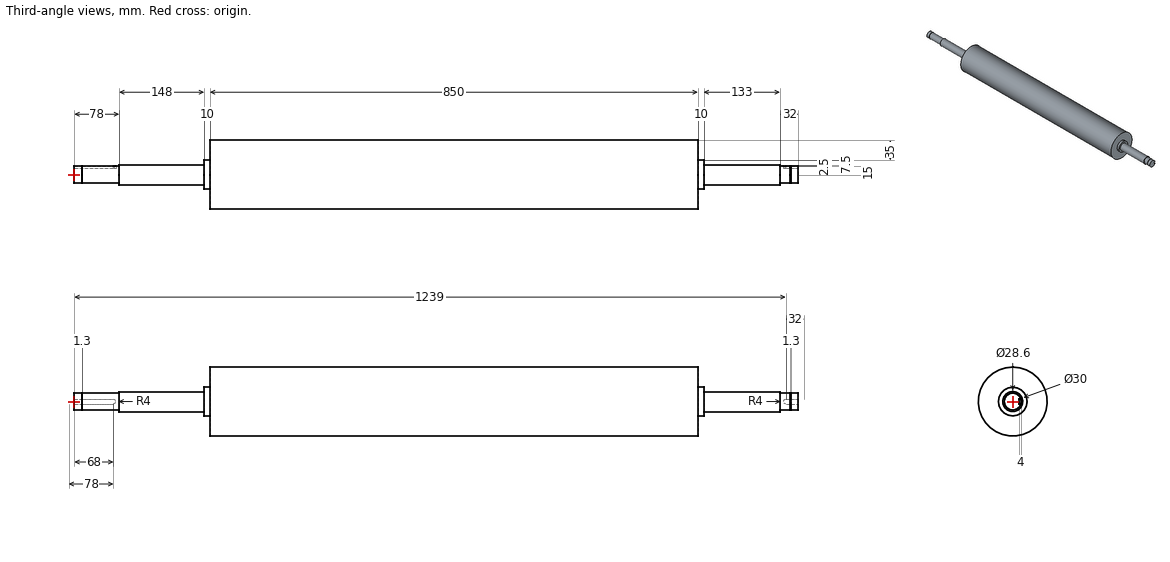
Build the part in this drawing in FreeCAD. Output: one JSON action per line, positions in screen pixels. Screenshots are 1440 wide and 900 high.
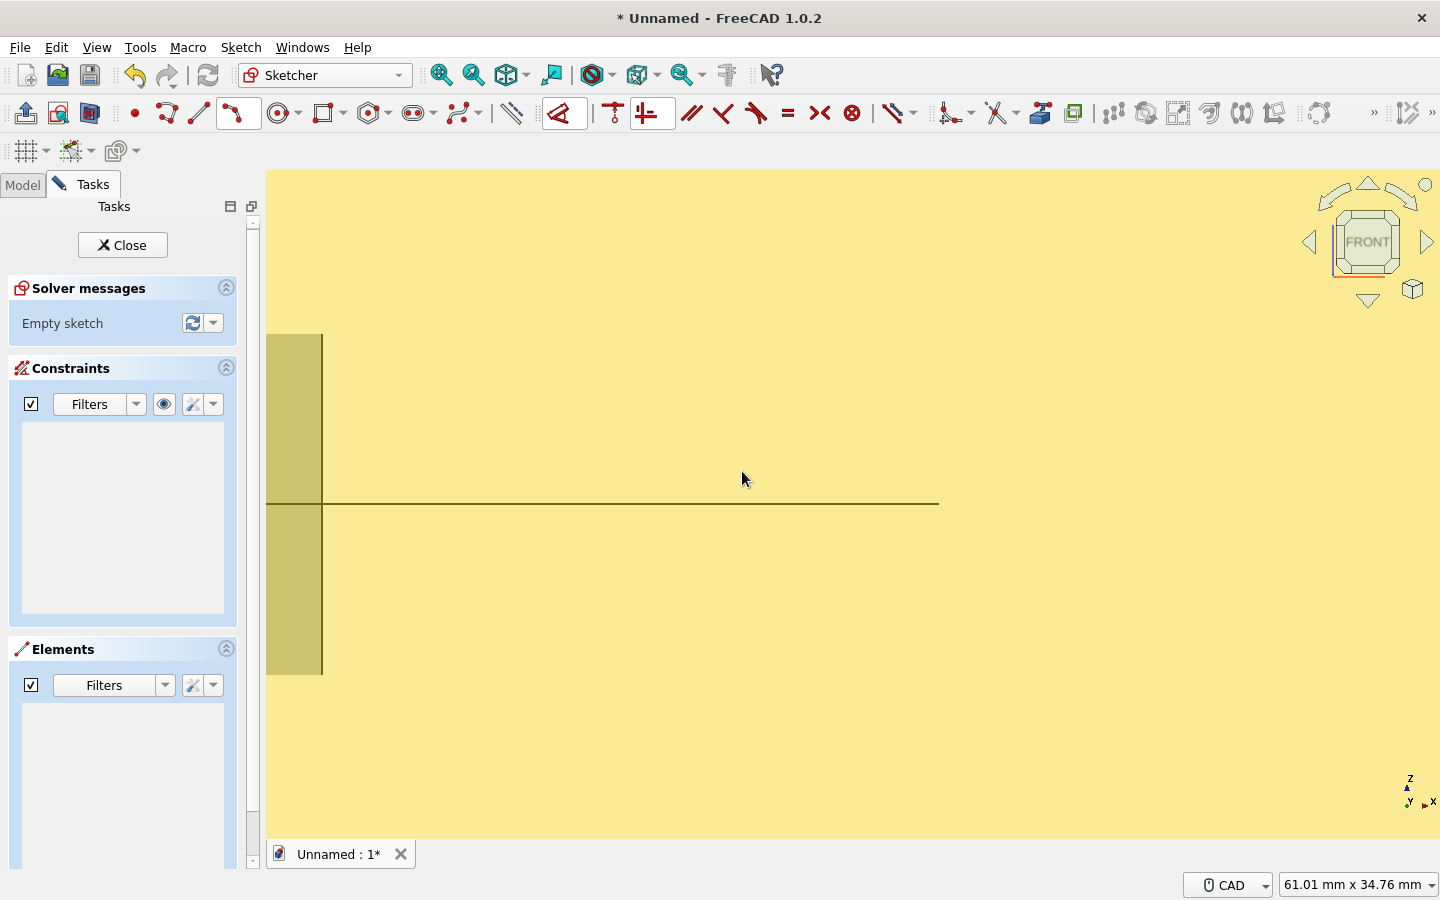
{"action": "left_click", "coordinate": [168, 114]}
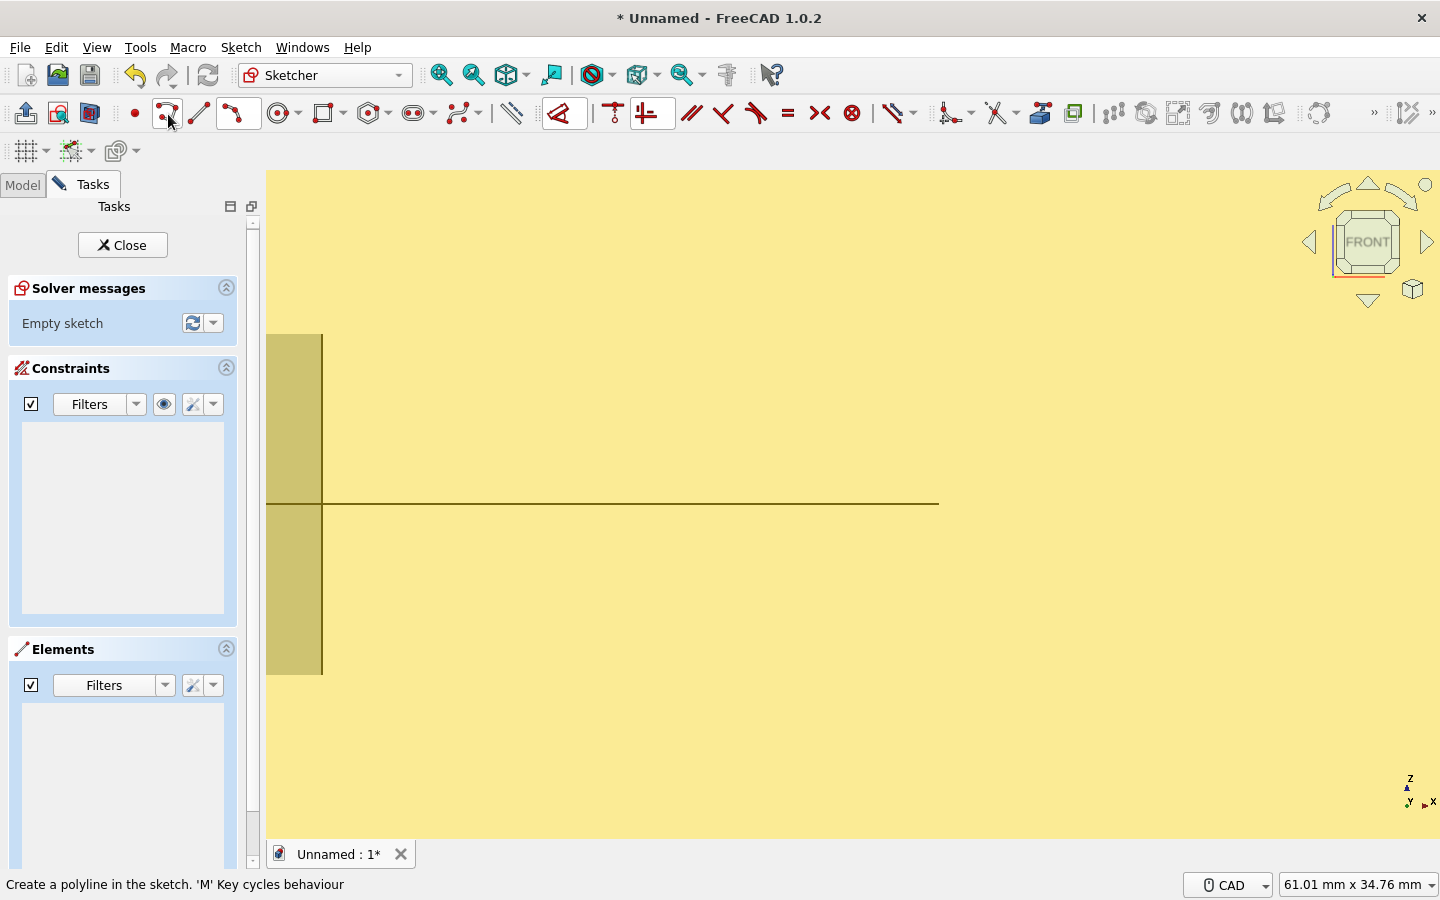
{"action": "left_click", "coordinate": [515, 427]}
{"action": "left_click", "coordinate": [1131, 427]}
{"action": "left_click", "coordinate": [1131, 581]}
{"action": "left_click", "coordinate": [515, 581]}
{"action": "right_click", "coordinate": [515, 581]}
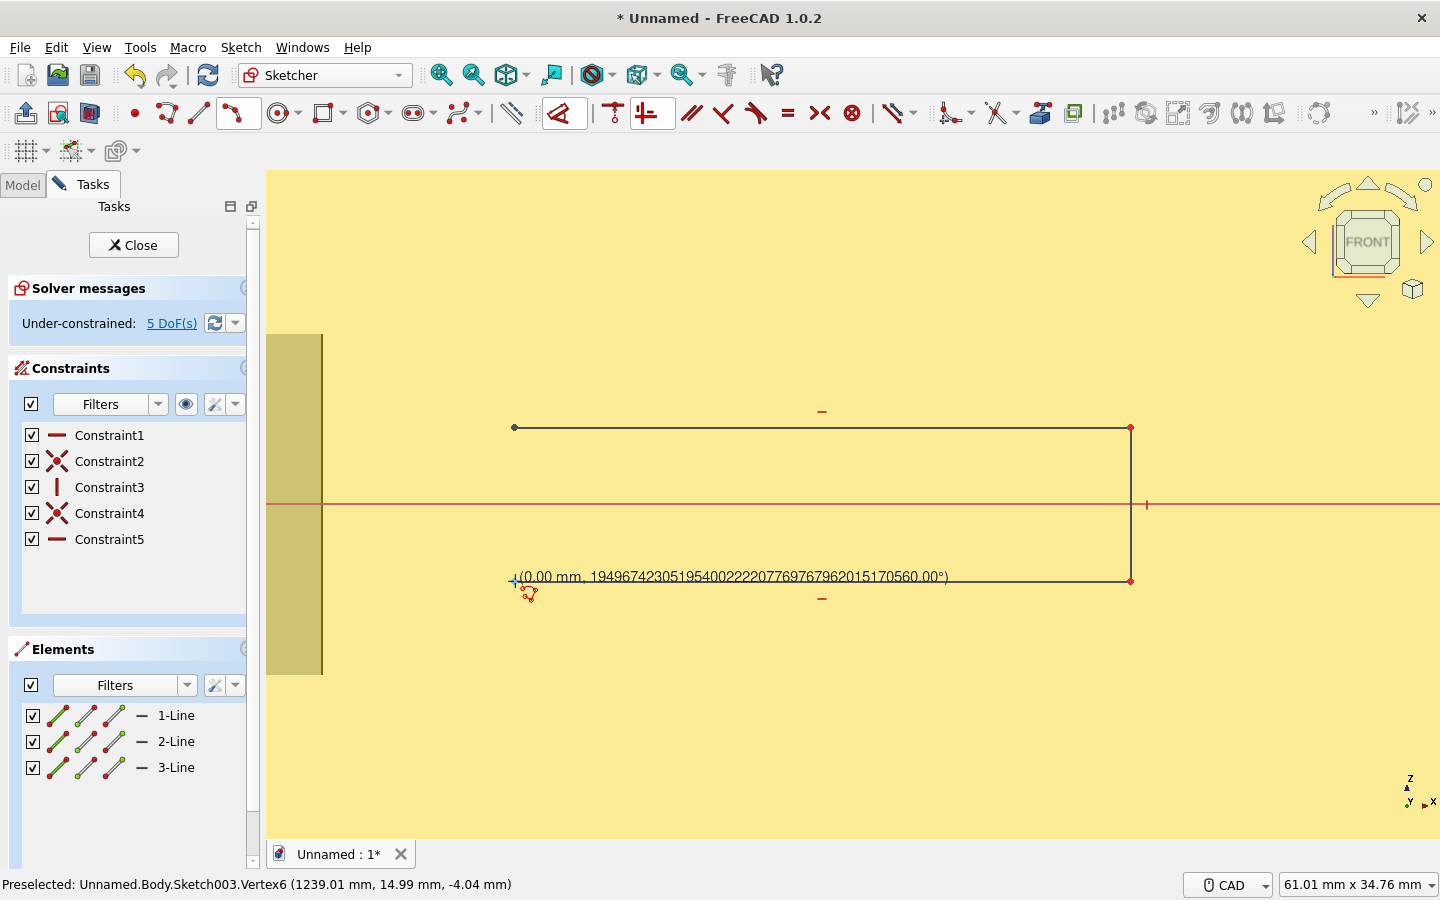
{"action": "left_click", "coordinate": [232, 114]}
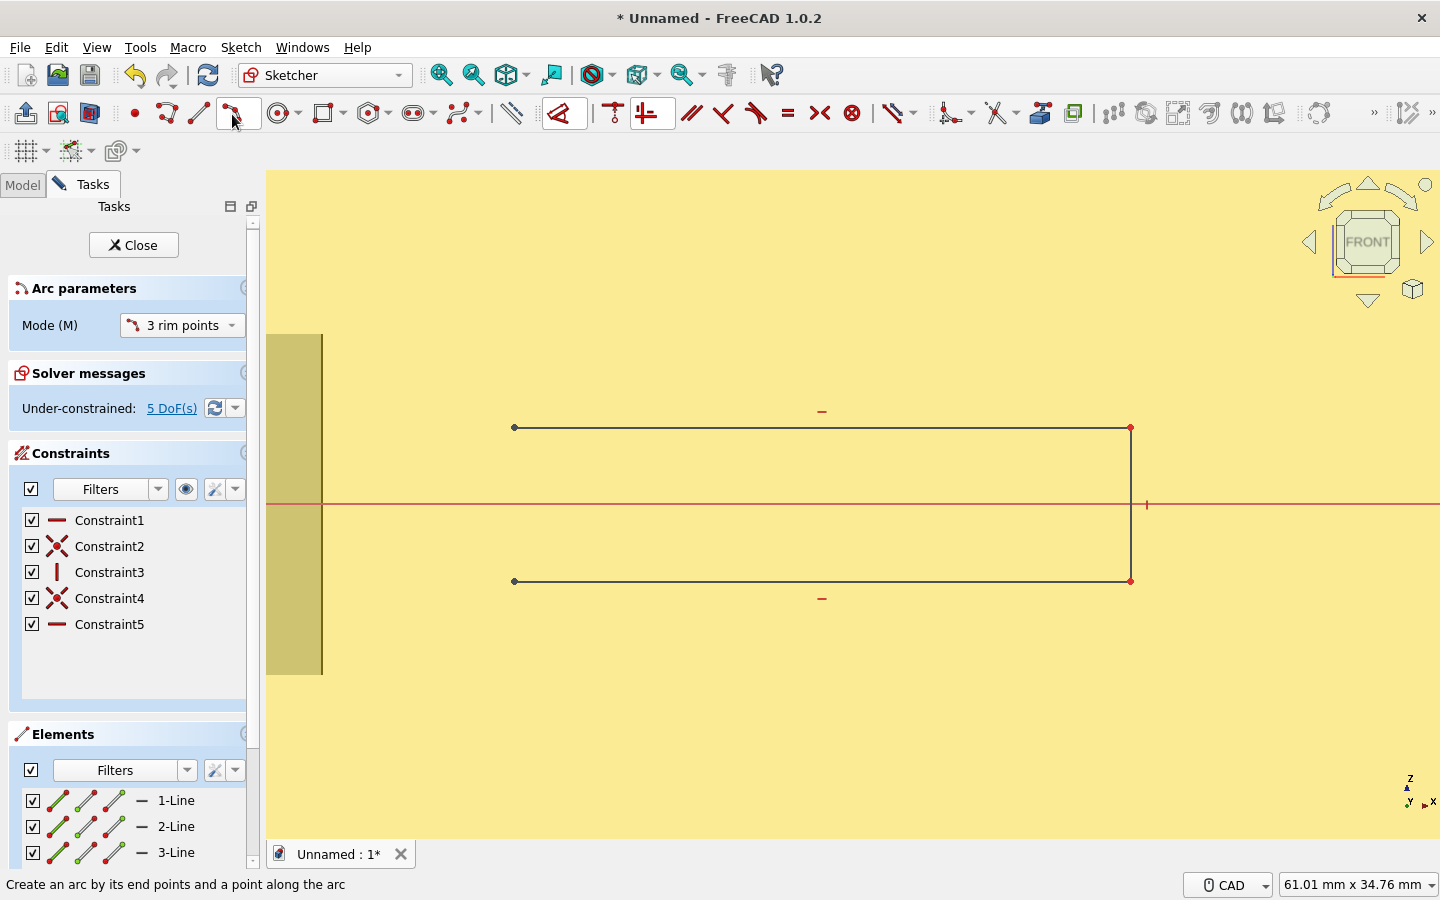
{"action": "left_click", "coordinate": [515, 582]}
{"action": "left_click", "coordinate": [515, 428]}
{"action": "left_click", "coordinate": [442, 481]}
{"action": "key", "text": "Escape"}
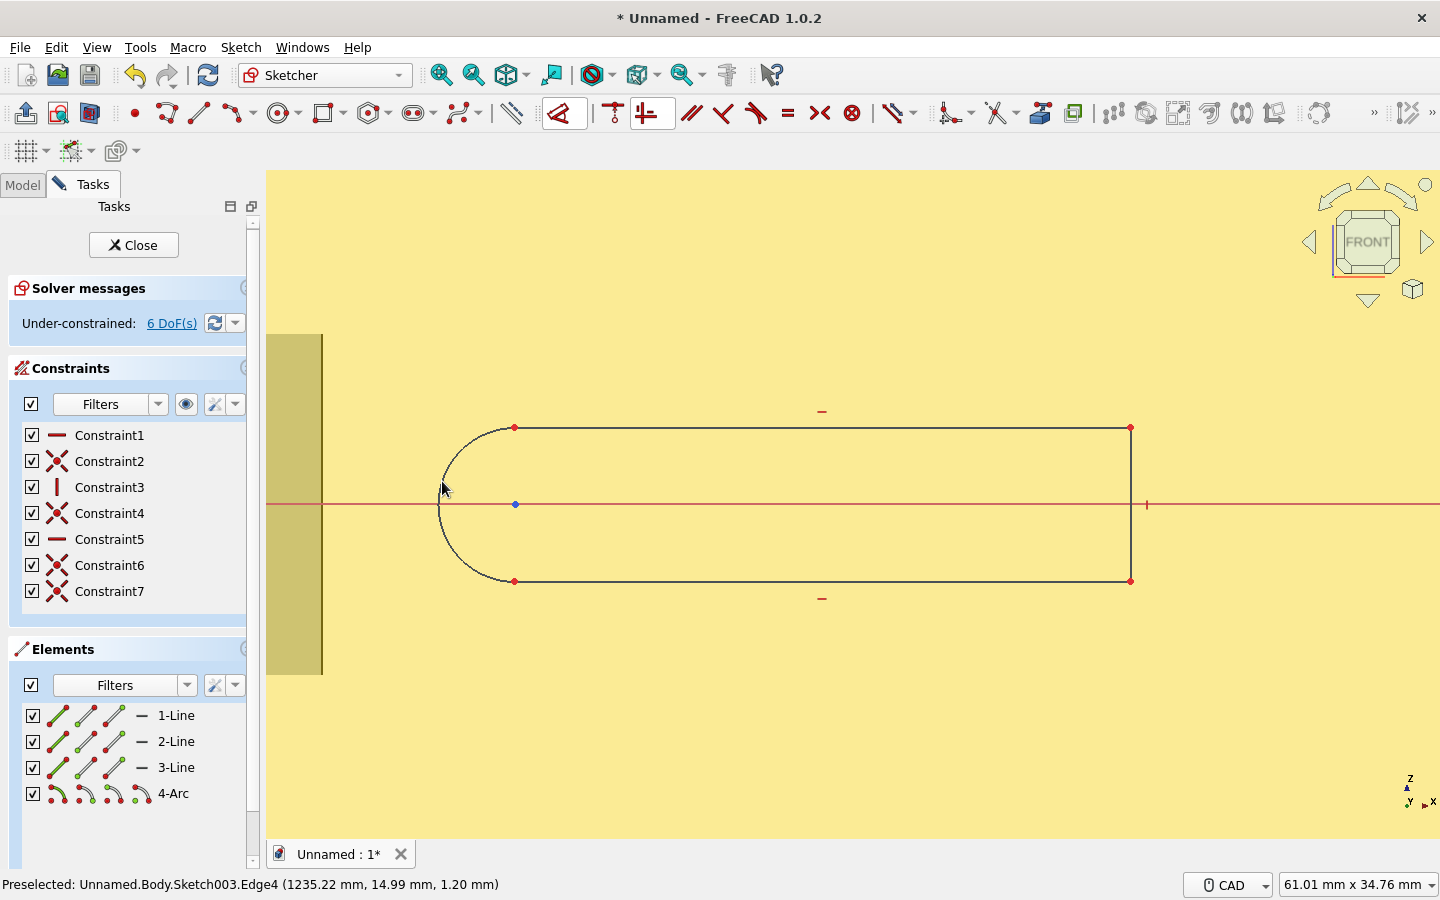
{"action": "left_click", "coordinate": [700, 428]}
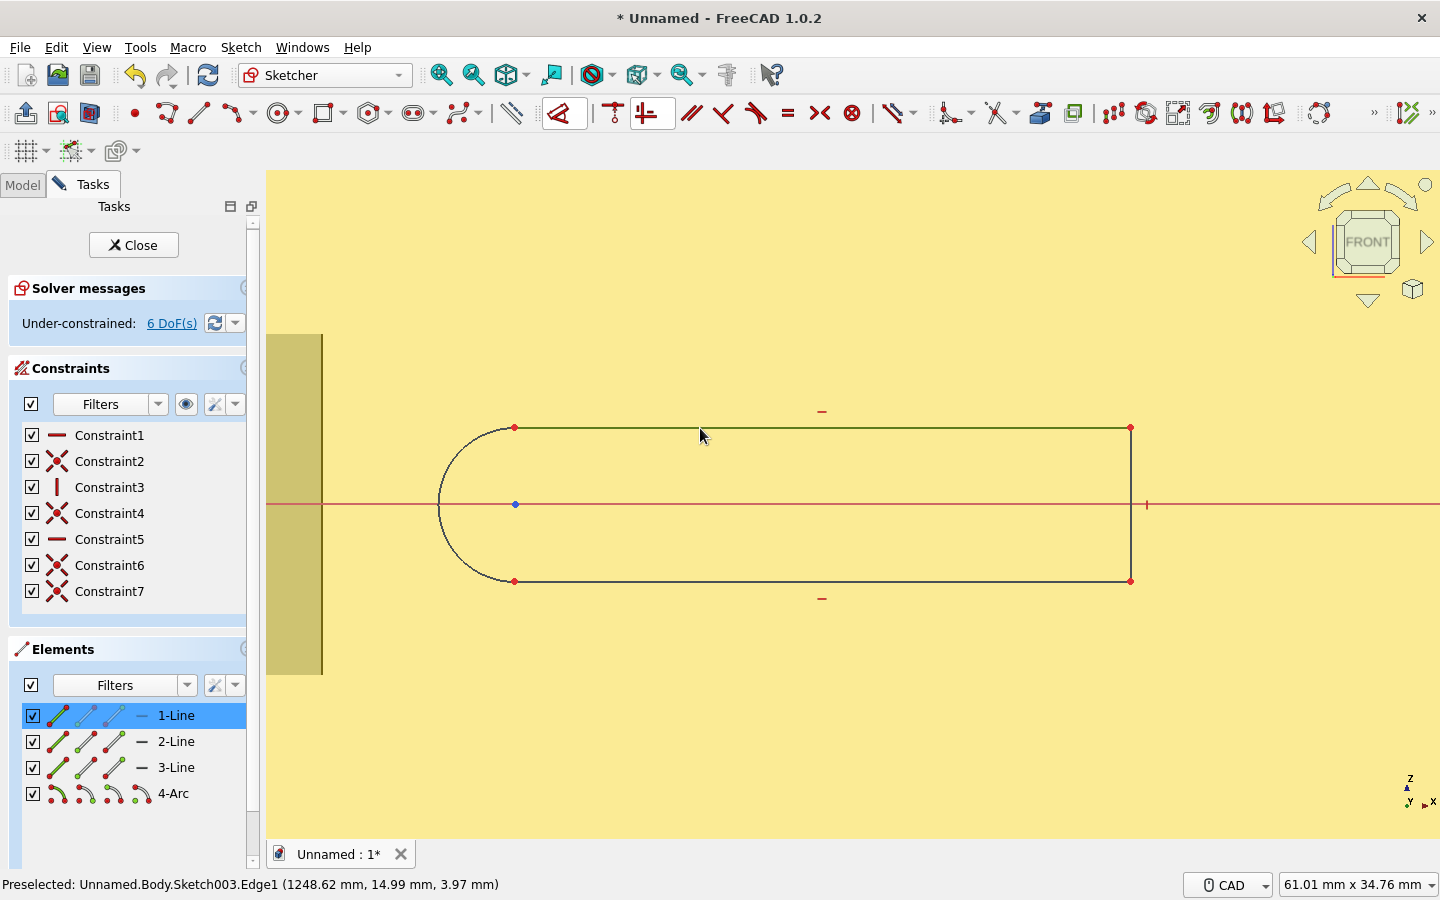
{"action": "left_click", "coordinate": [453, 460]}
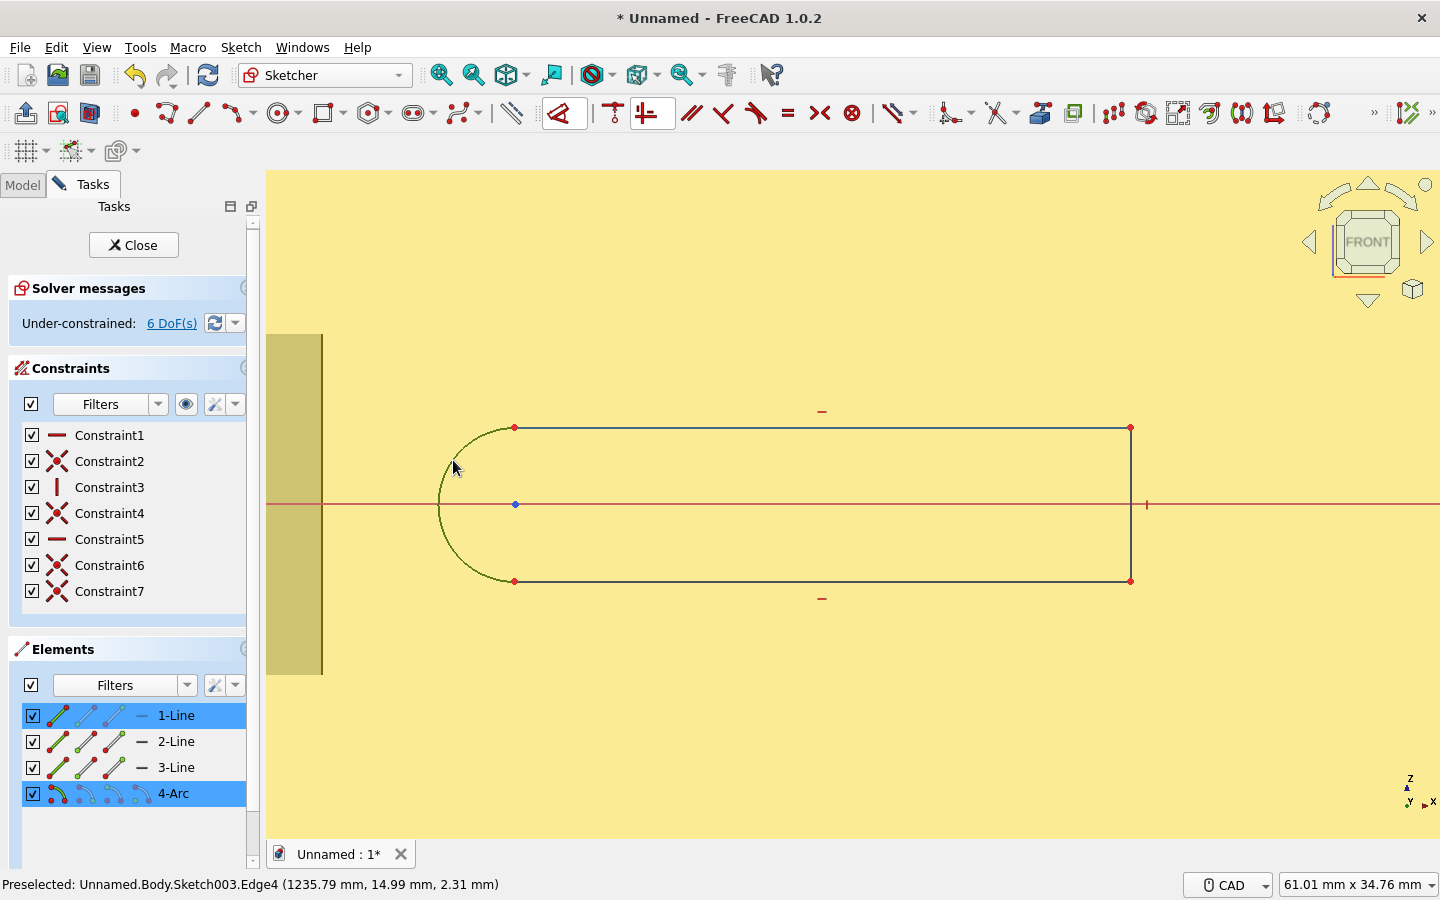
{"action": "left_click", "coordinate": [756, 114]}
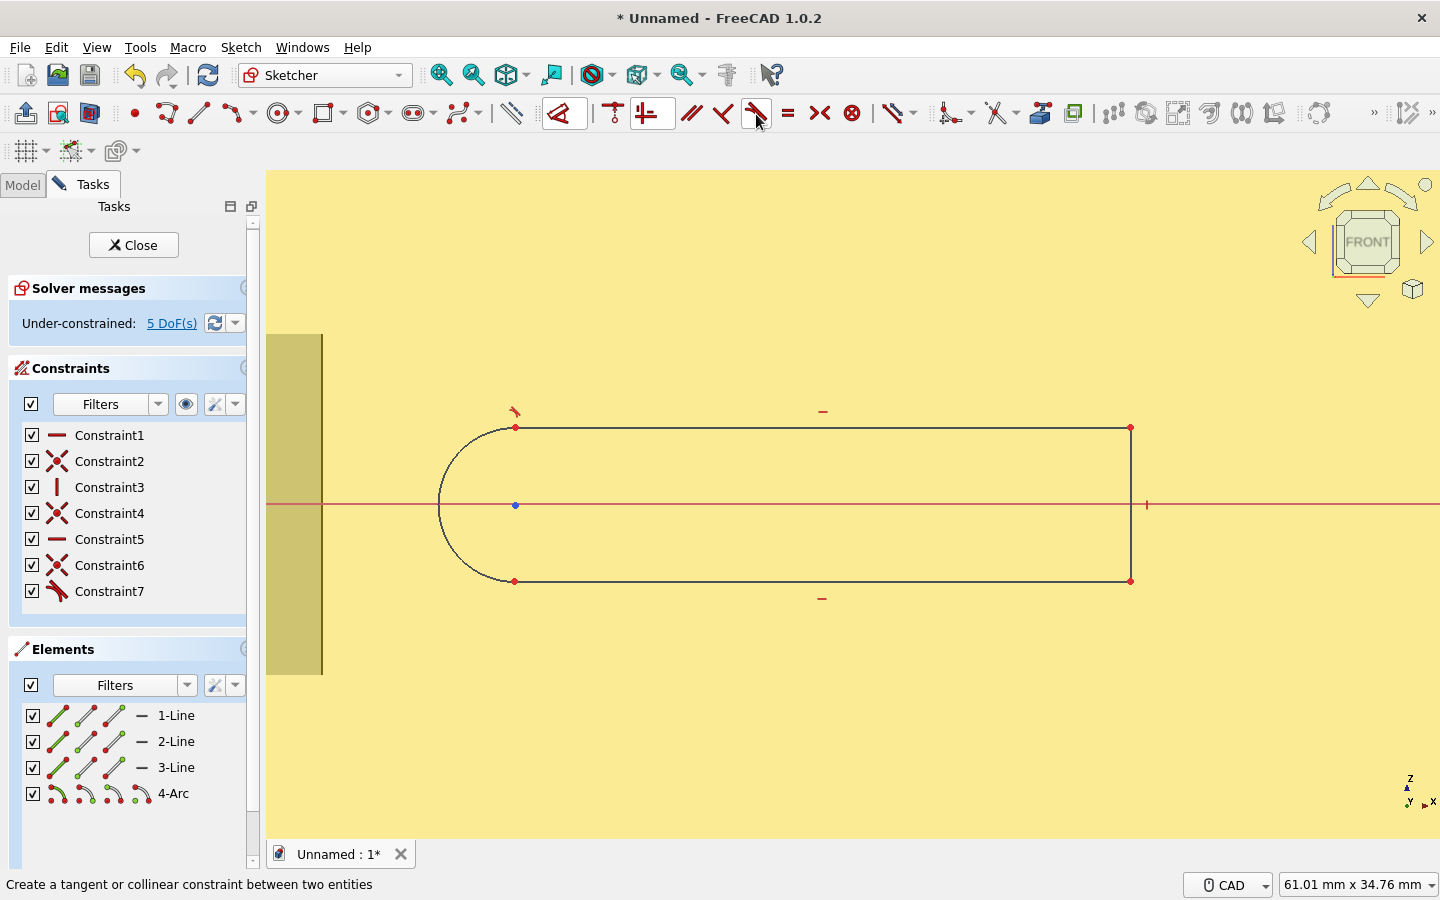
{"action": "left_click", "coordinate": [946, 582]}